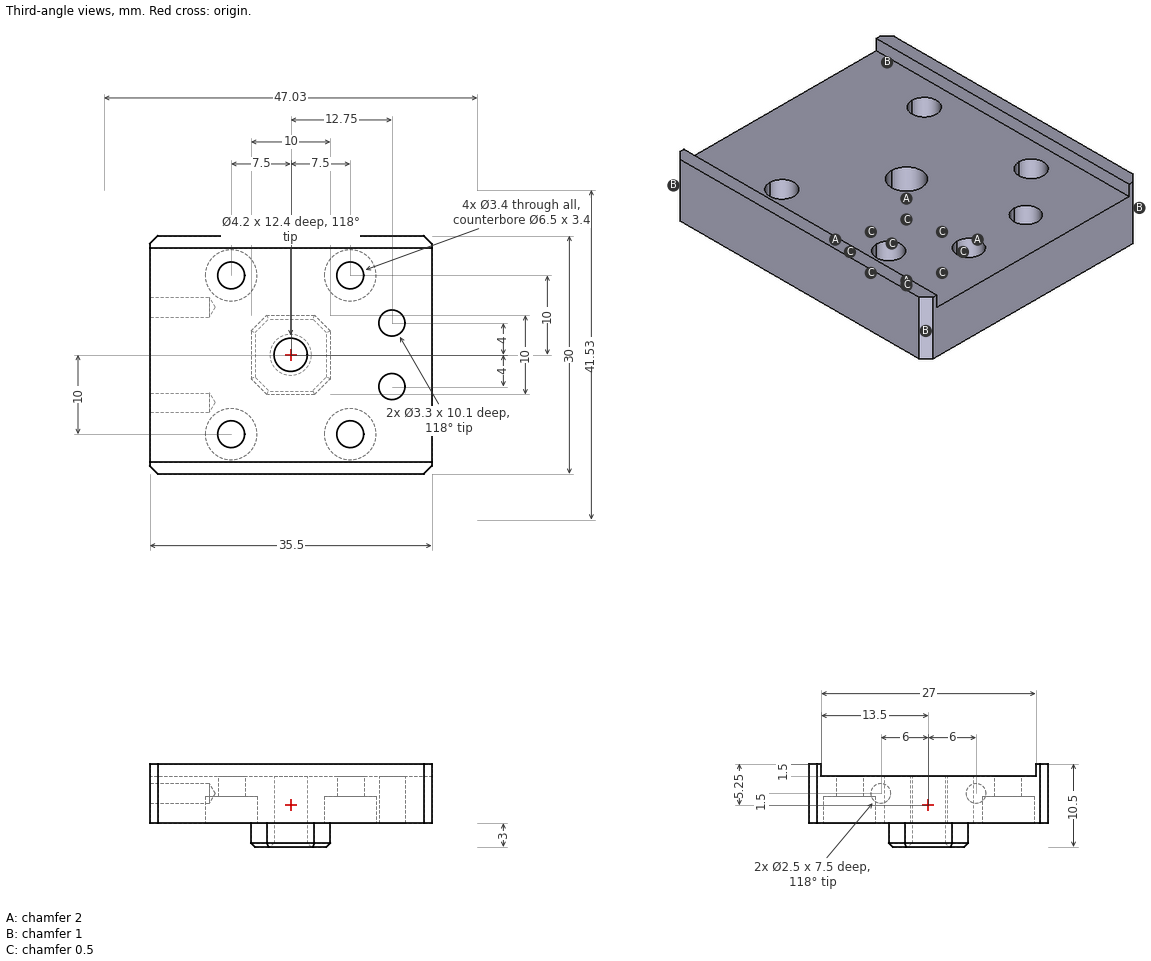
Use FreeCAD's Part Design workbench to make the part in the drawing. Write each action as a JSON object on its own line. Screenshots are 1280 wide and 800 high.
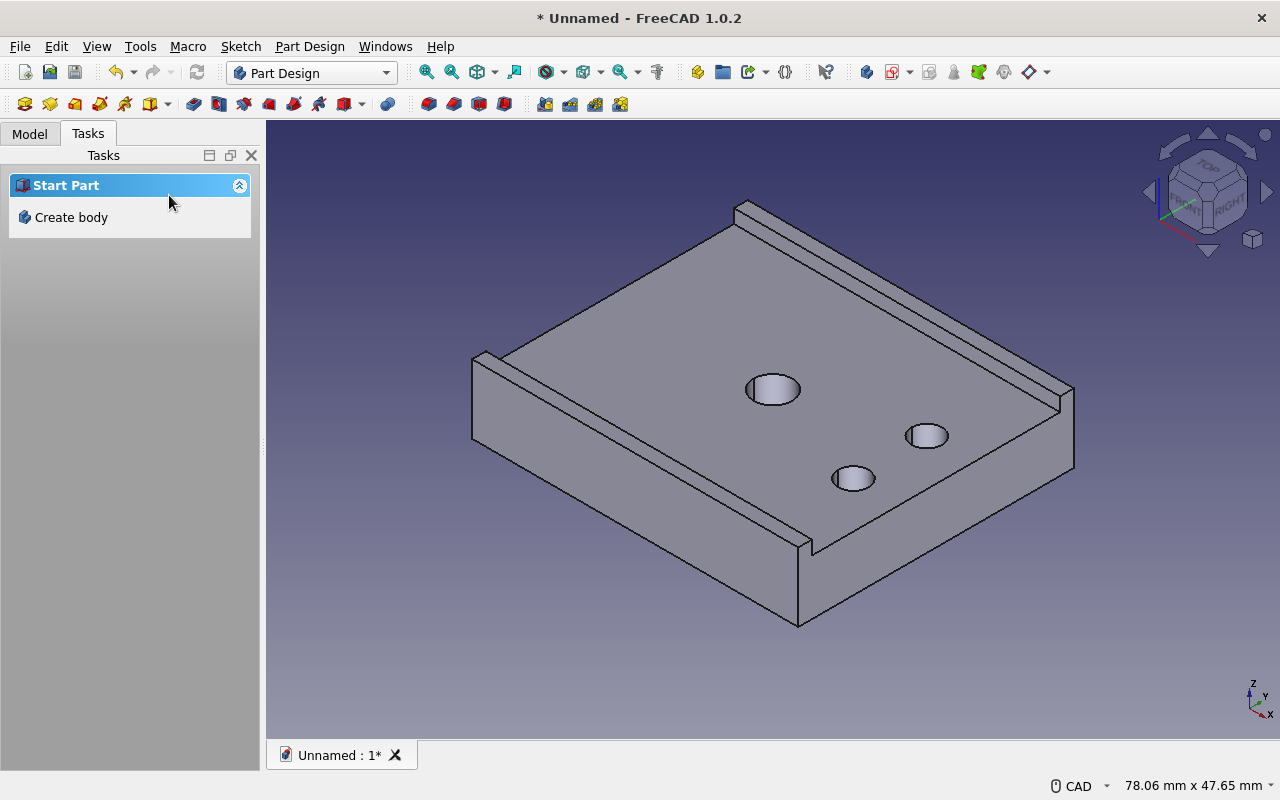
{"action": "left_click", "coordinate": [798, 586]}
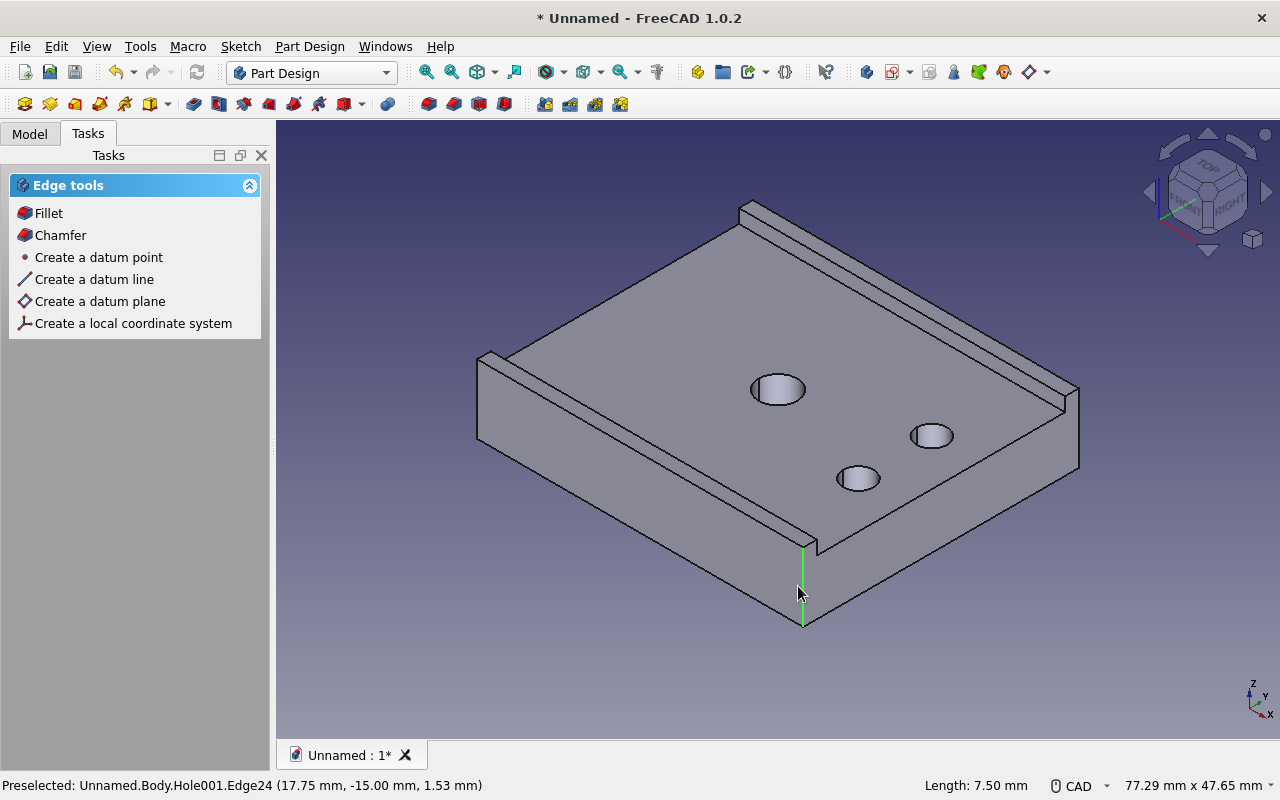
{"action": "key", "text": "2"}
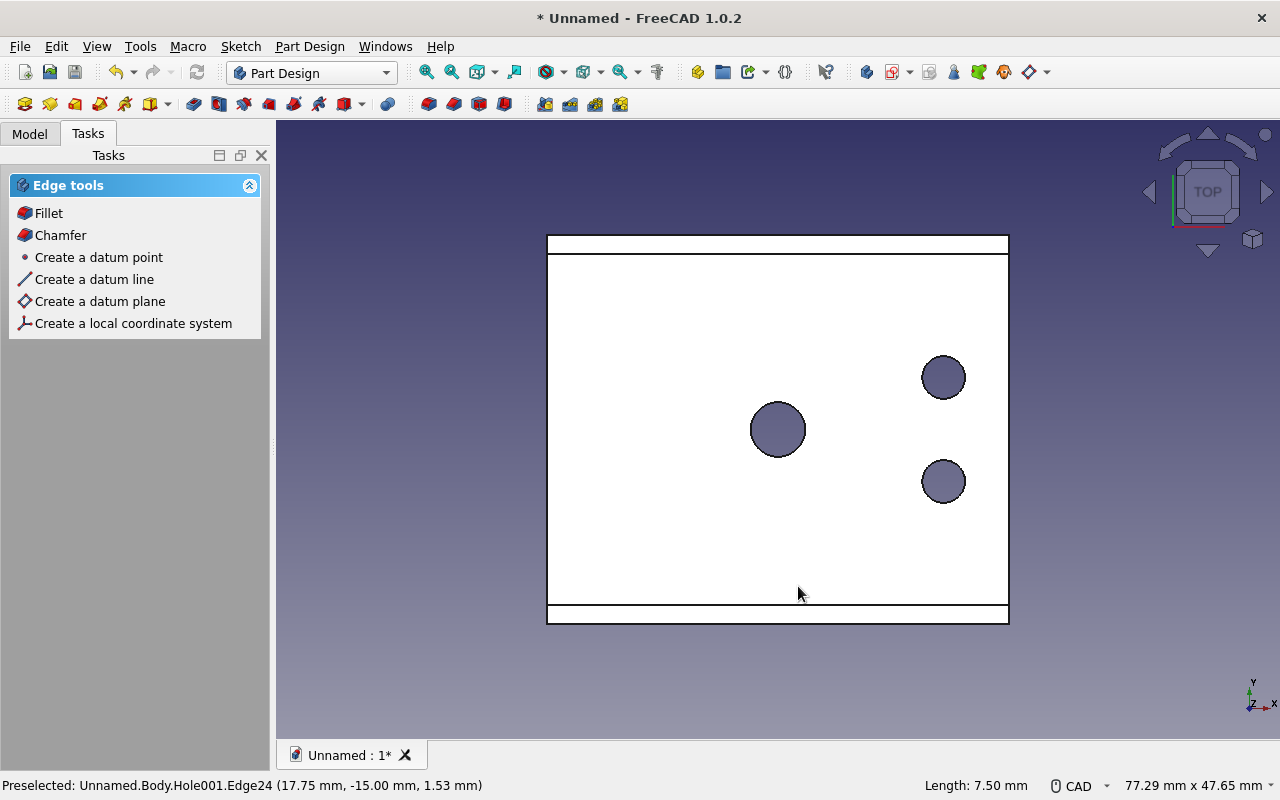
{"action": "key", "text": "1"}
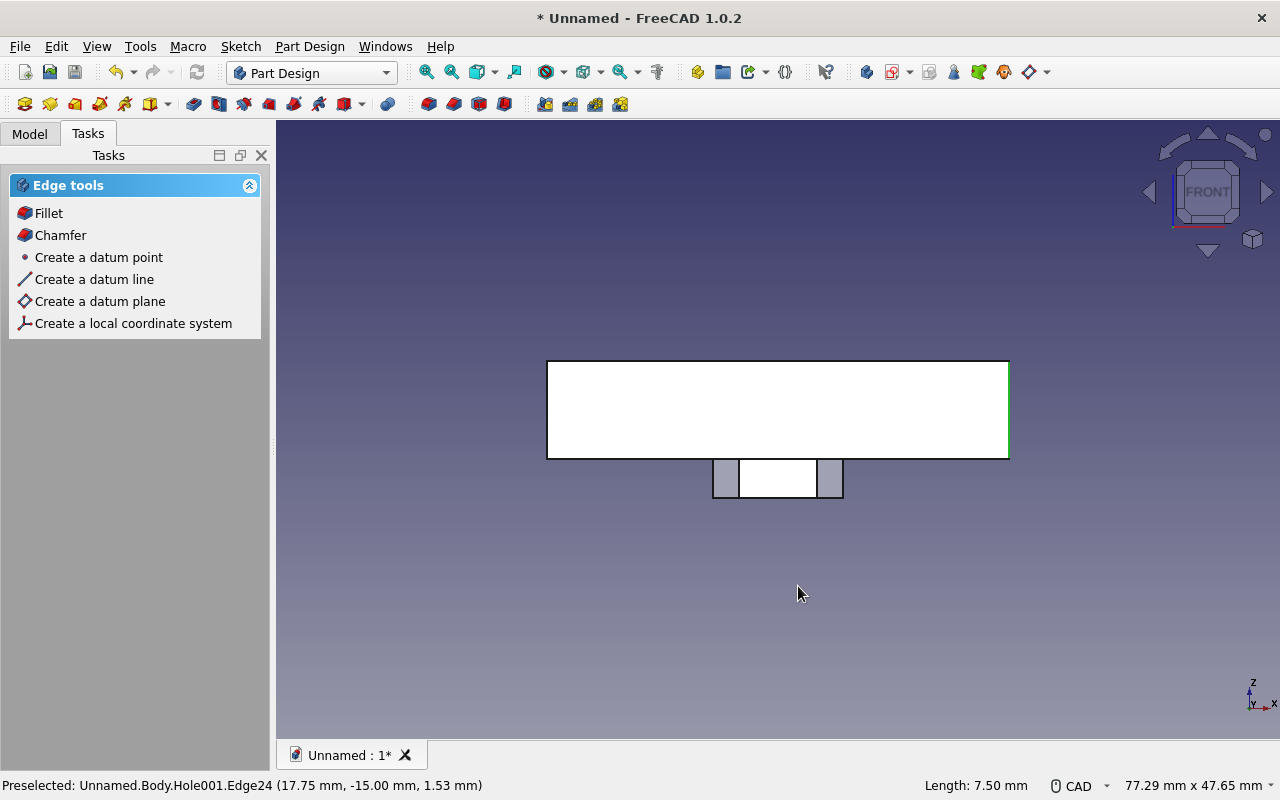
{"action": "left_click", "coordinate": [547, 409], "text": "ctrl"}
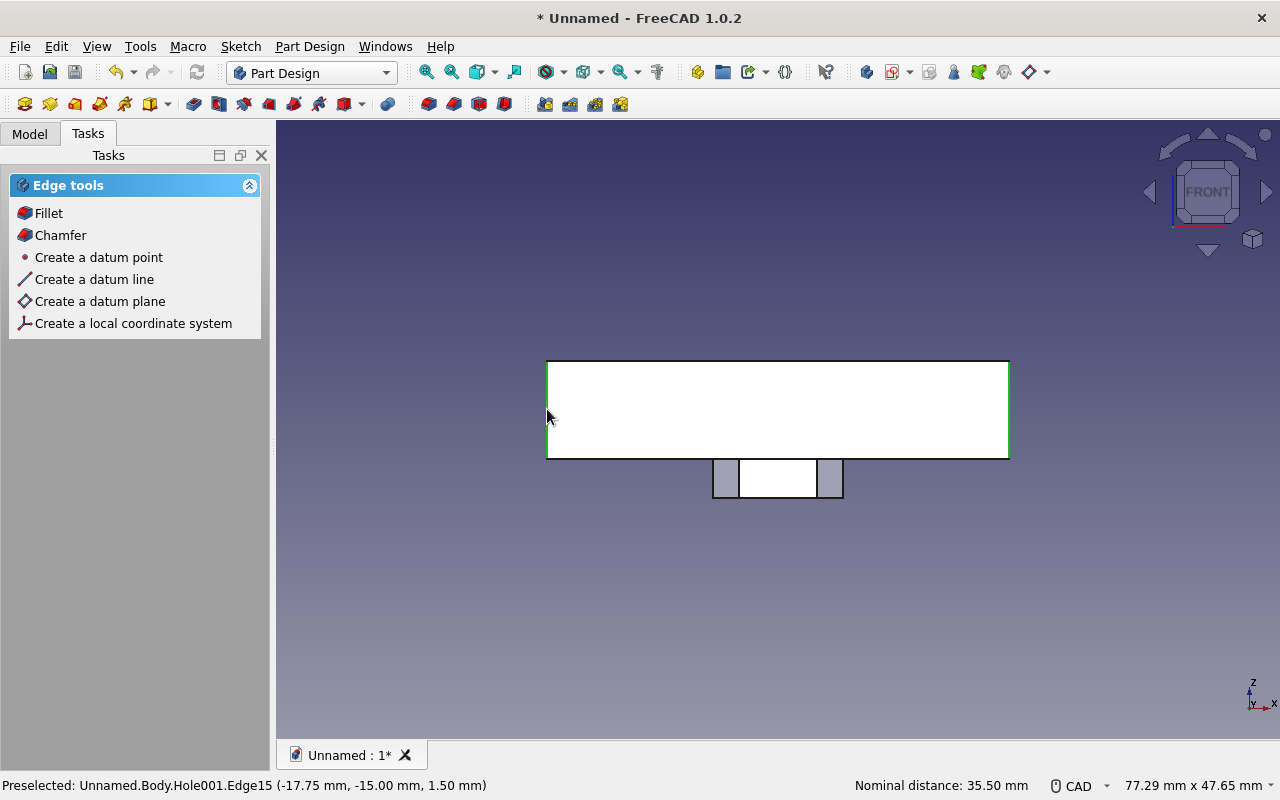
{"action": "key", "text": "3"}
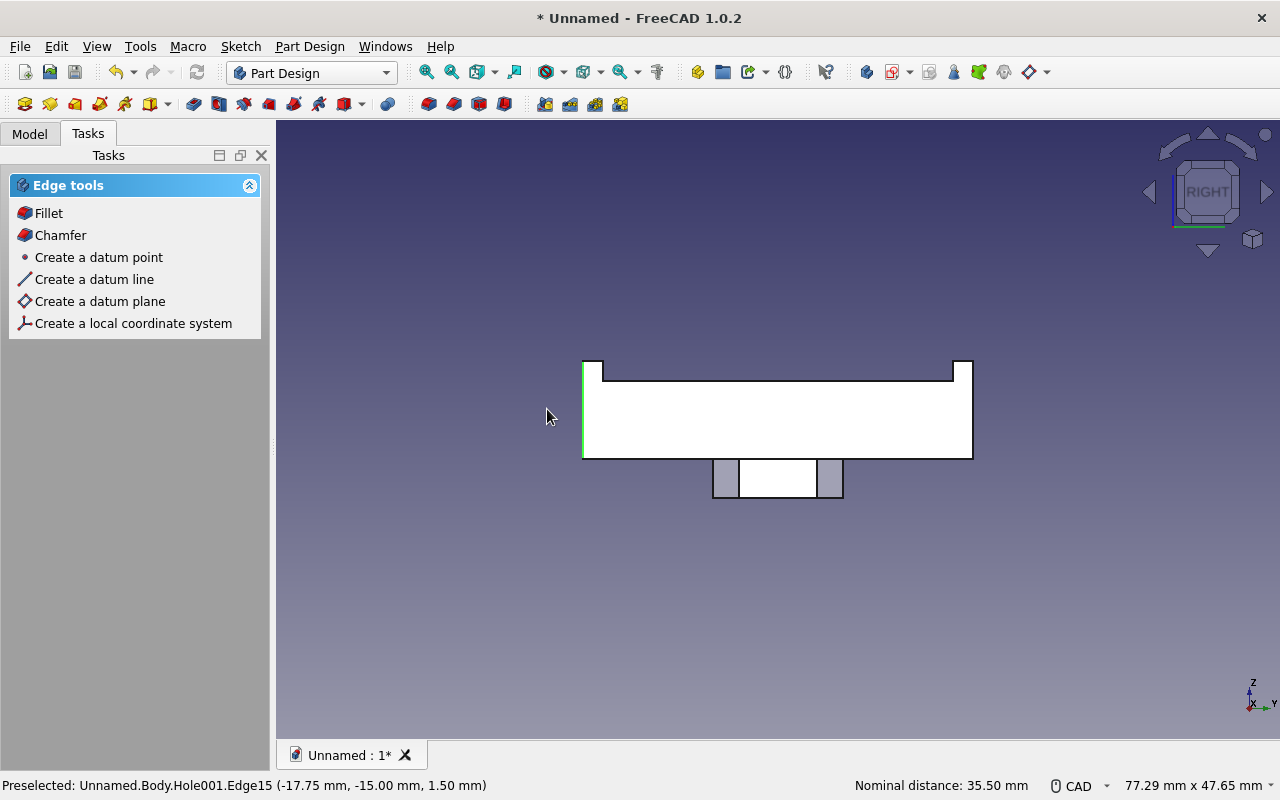
{"action": "key", "text": "v f"}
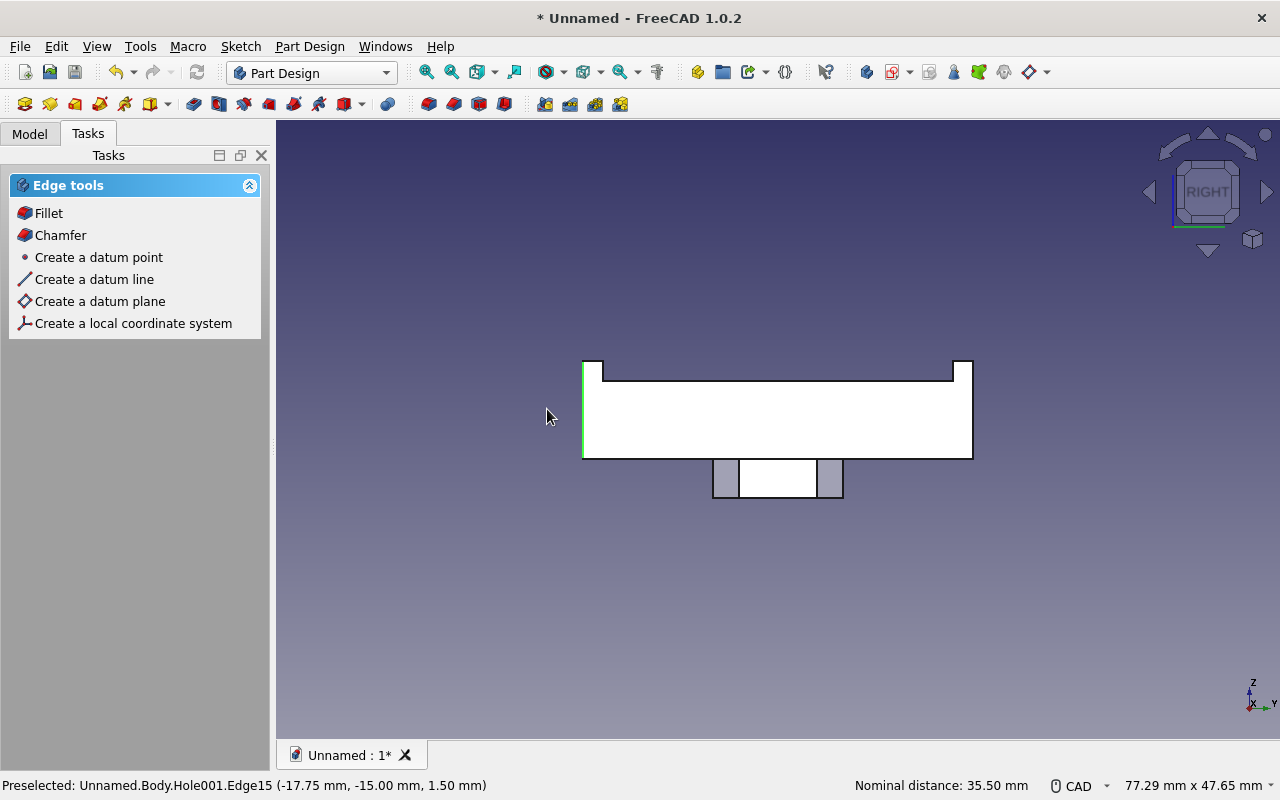
{"action": "left_click", "coordinate": [973, 409], "text": "ctrl"}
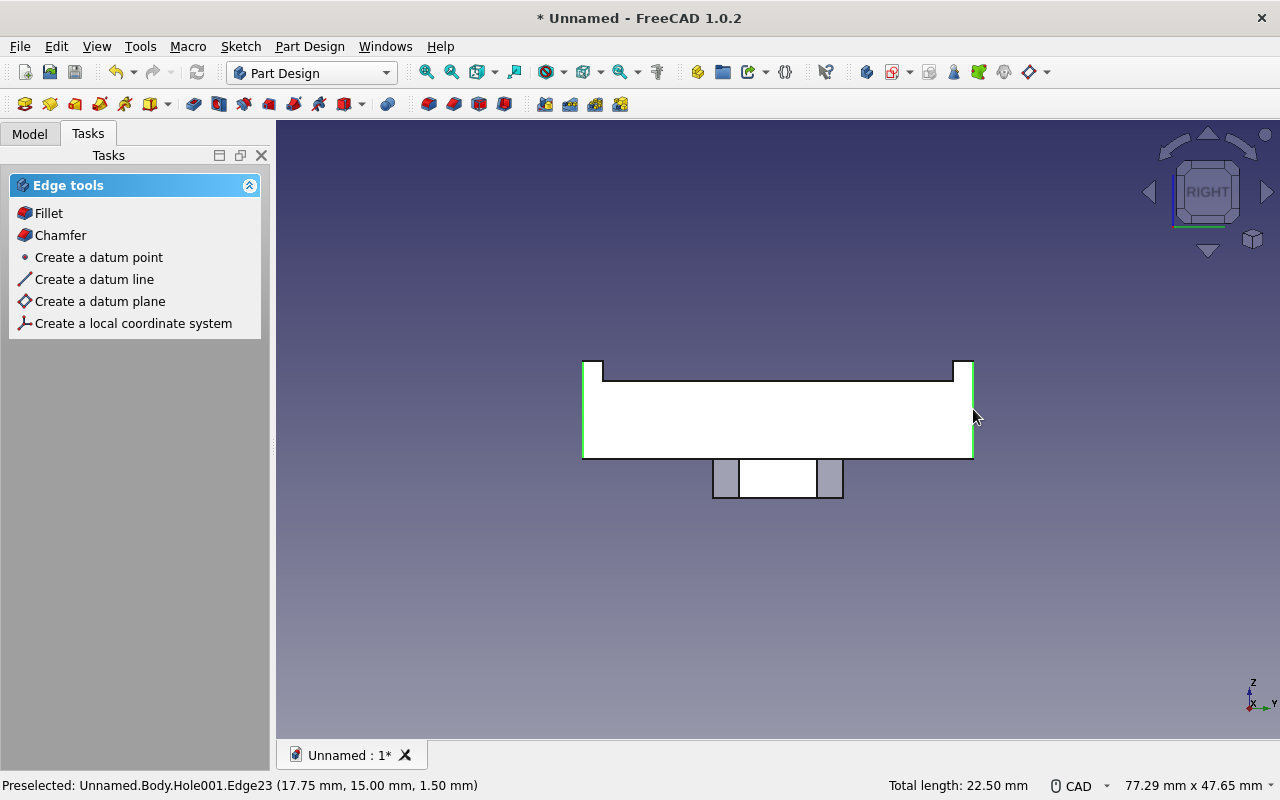
{"action": "key", "text": "5"}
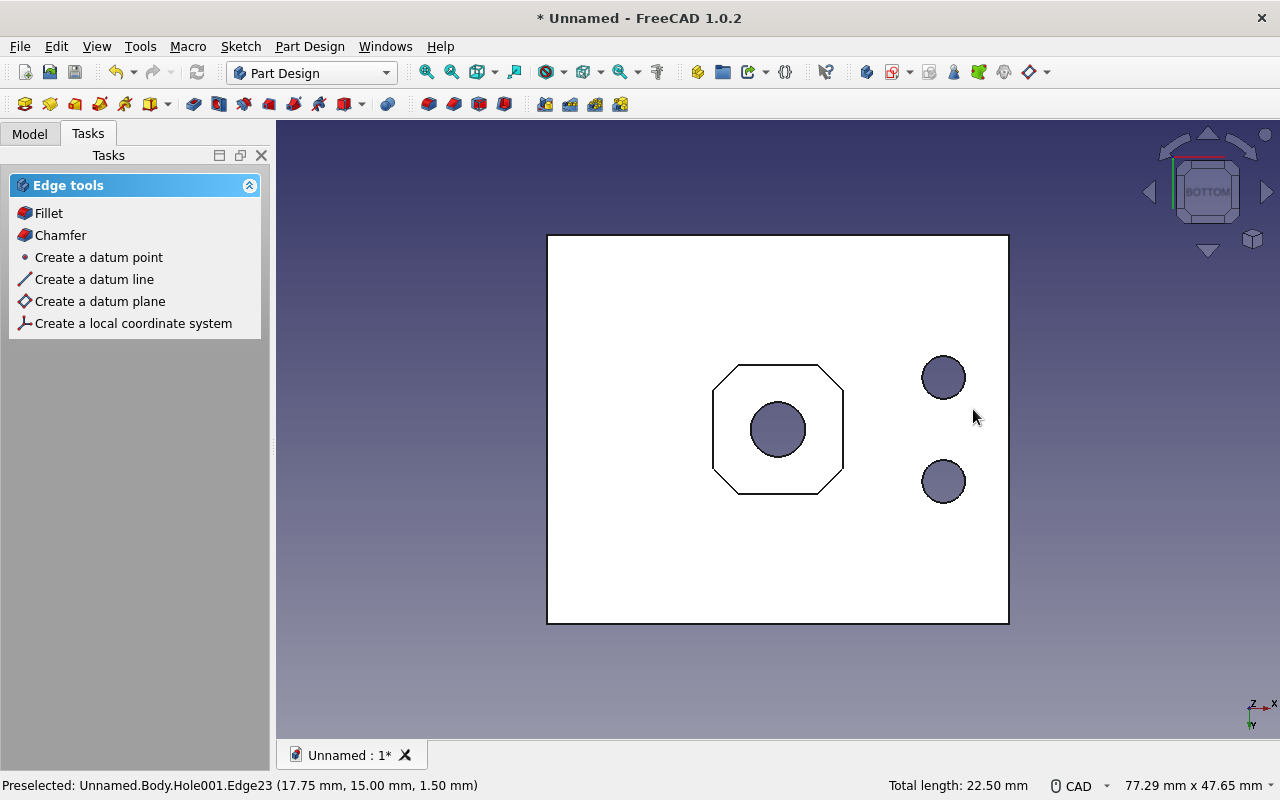
{"action": "key", "text": "4"}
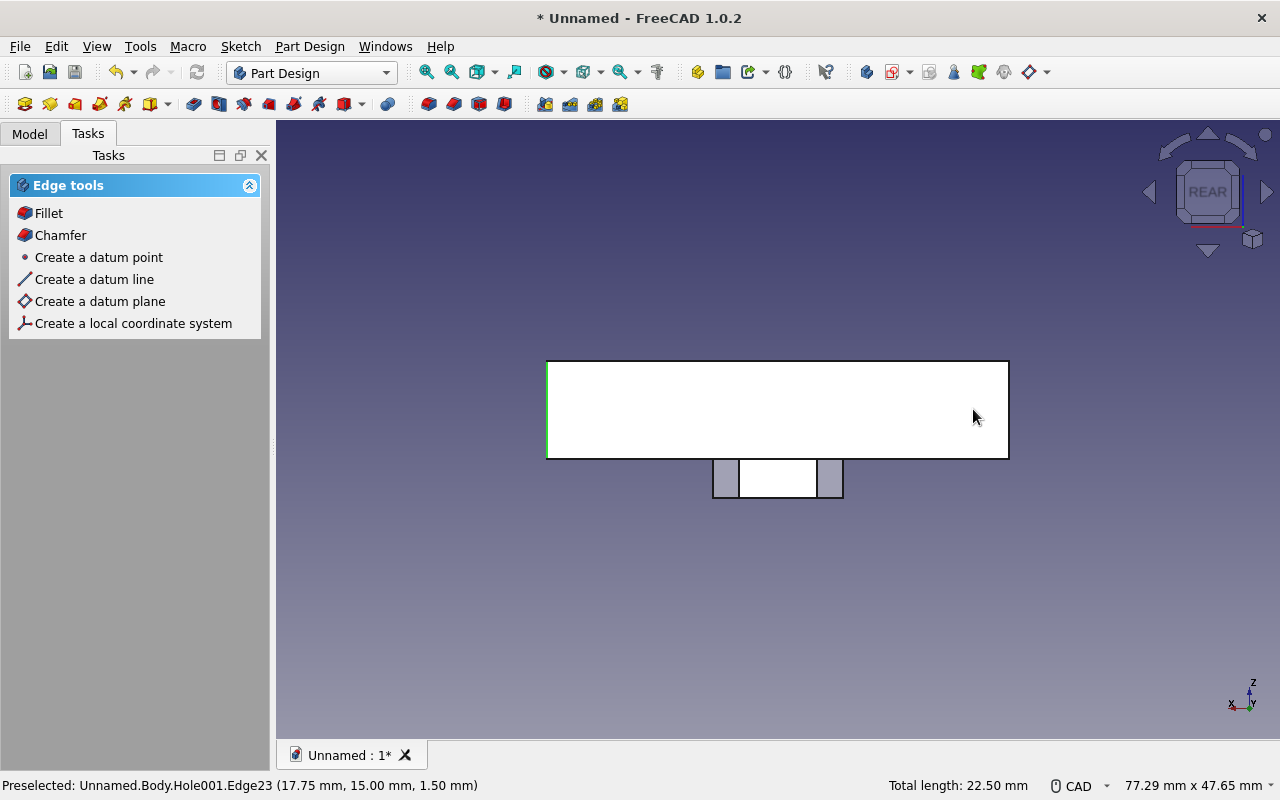
{"action": "left_click", "coordinate": [1009, 409], "text": "ctrl"}